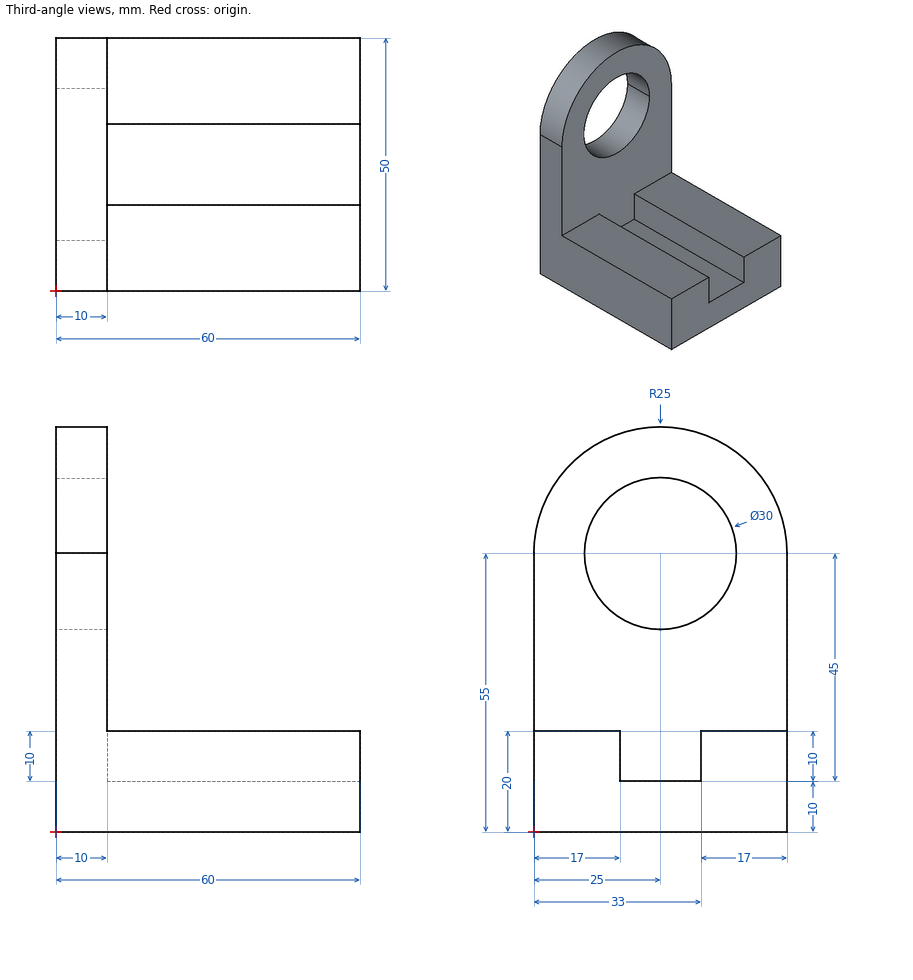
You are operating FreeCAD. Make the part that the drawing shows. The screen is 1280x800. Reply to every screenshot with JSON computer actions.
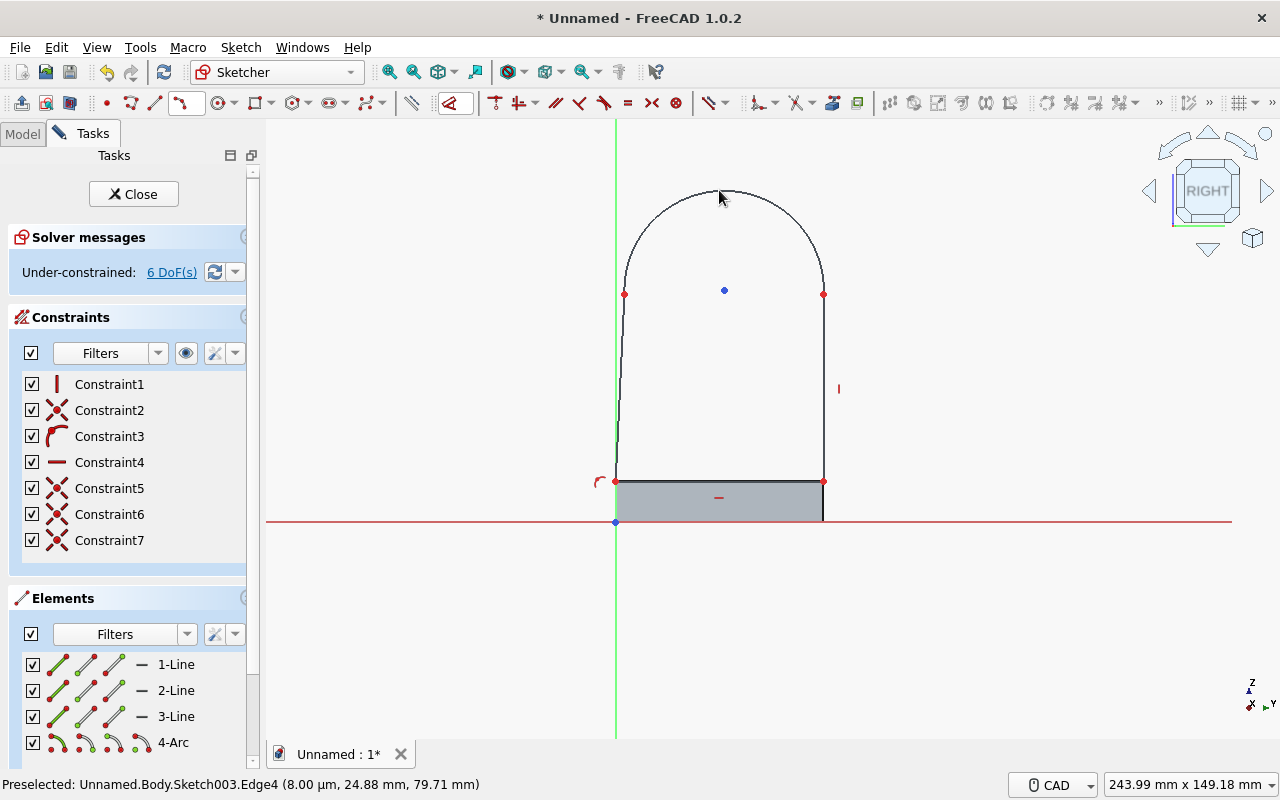
{"action": "left_click", "coordinate": [824, 351]}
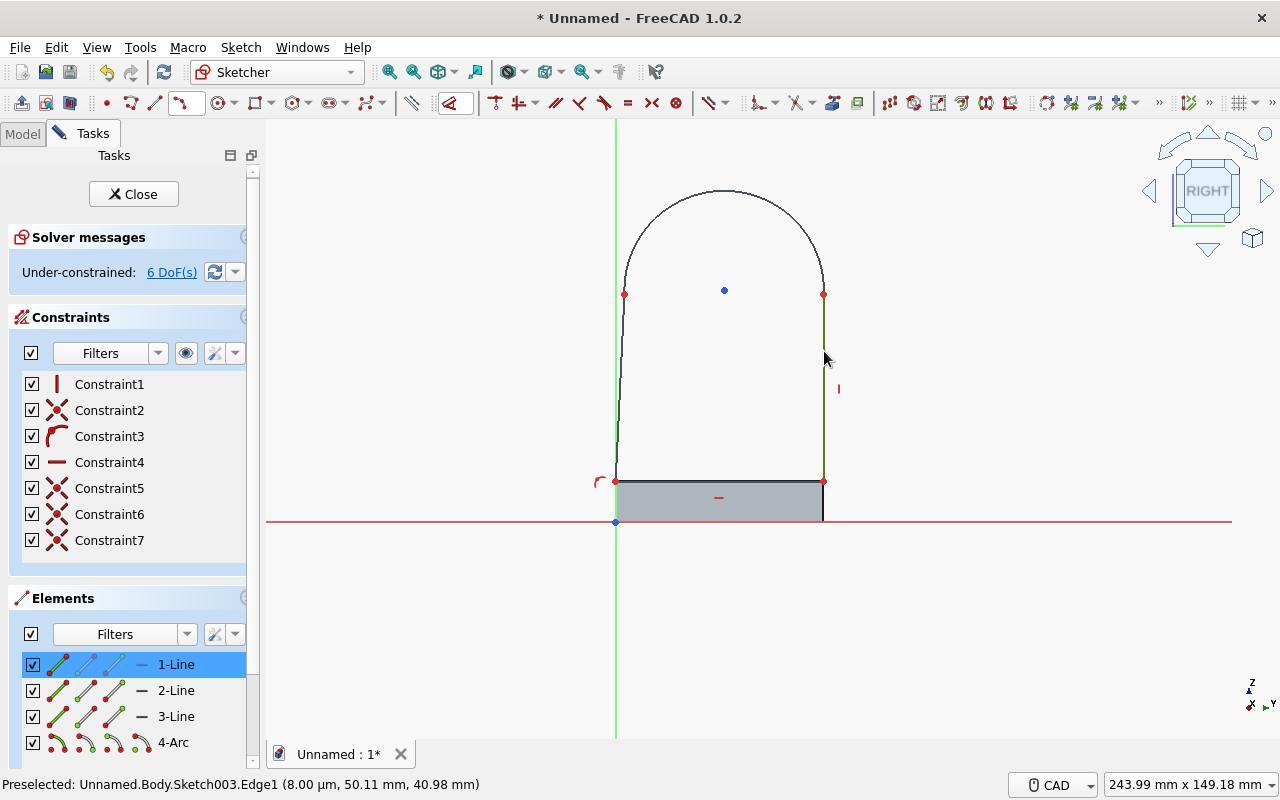
{"action": "left_click", "coordinate": [784, 211]}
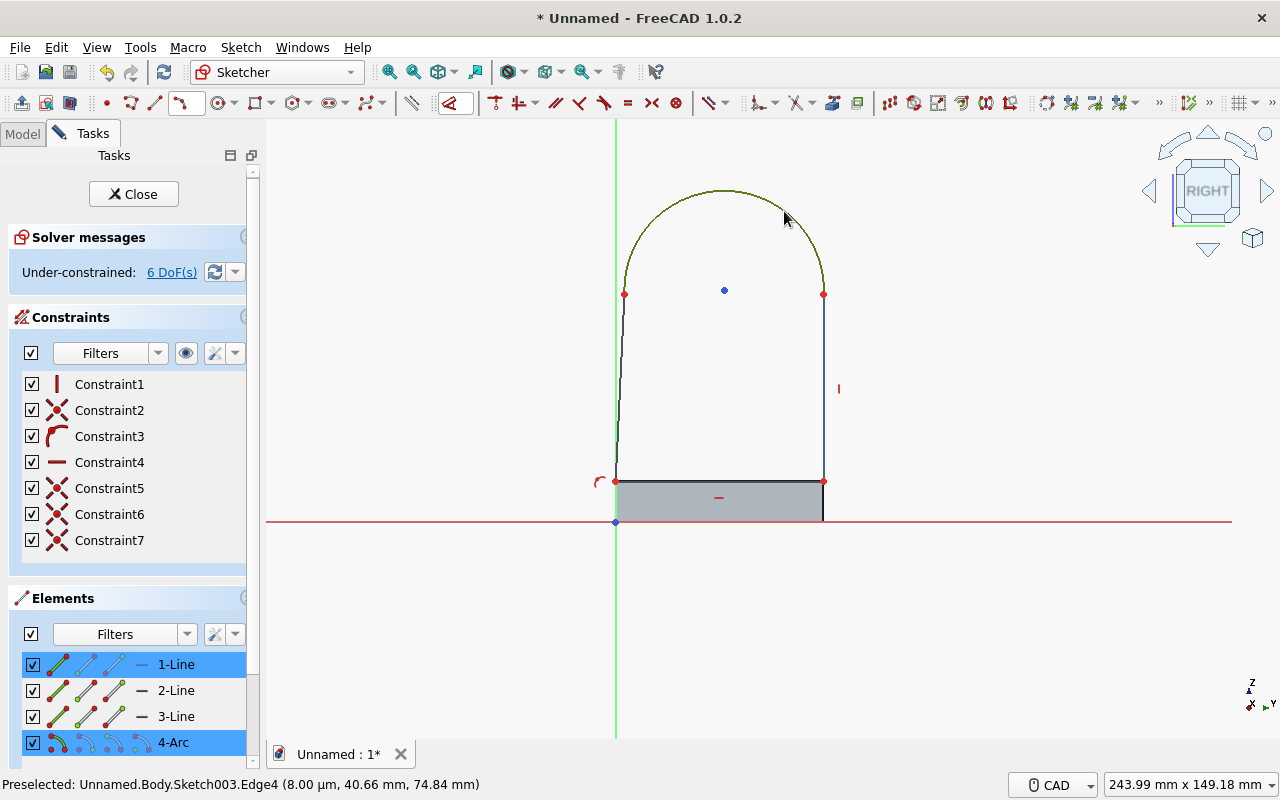
{"action": "left_click", "coordinate": [604, 104]}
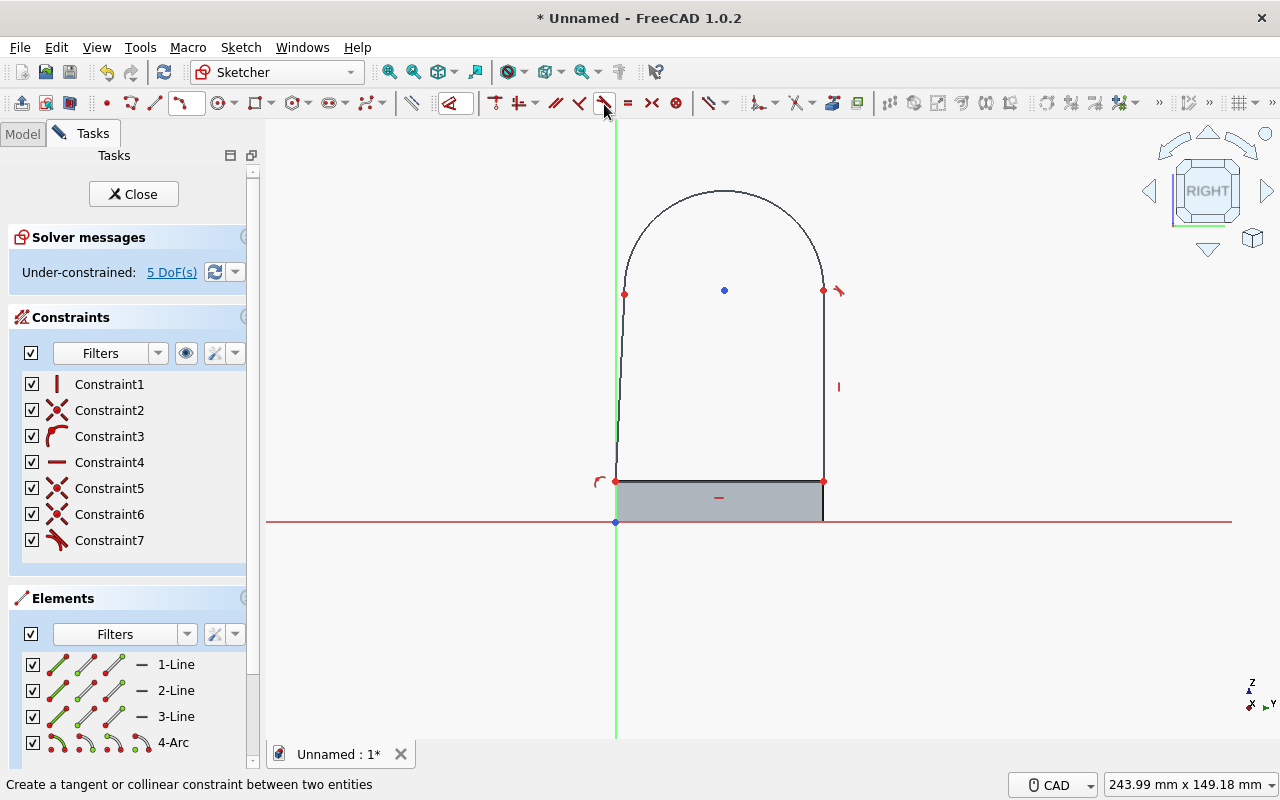
{"action": "left_click", "coordinate": [618, 426]}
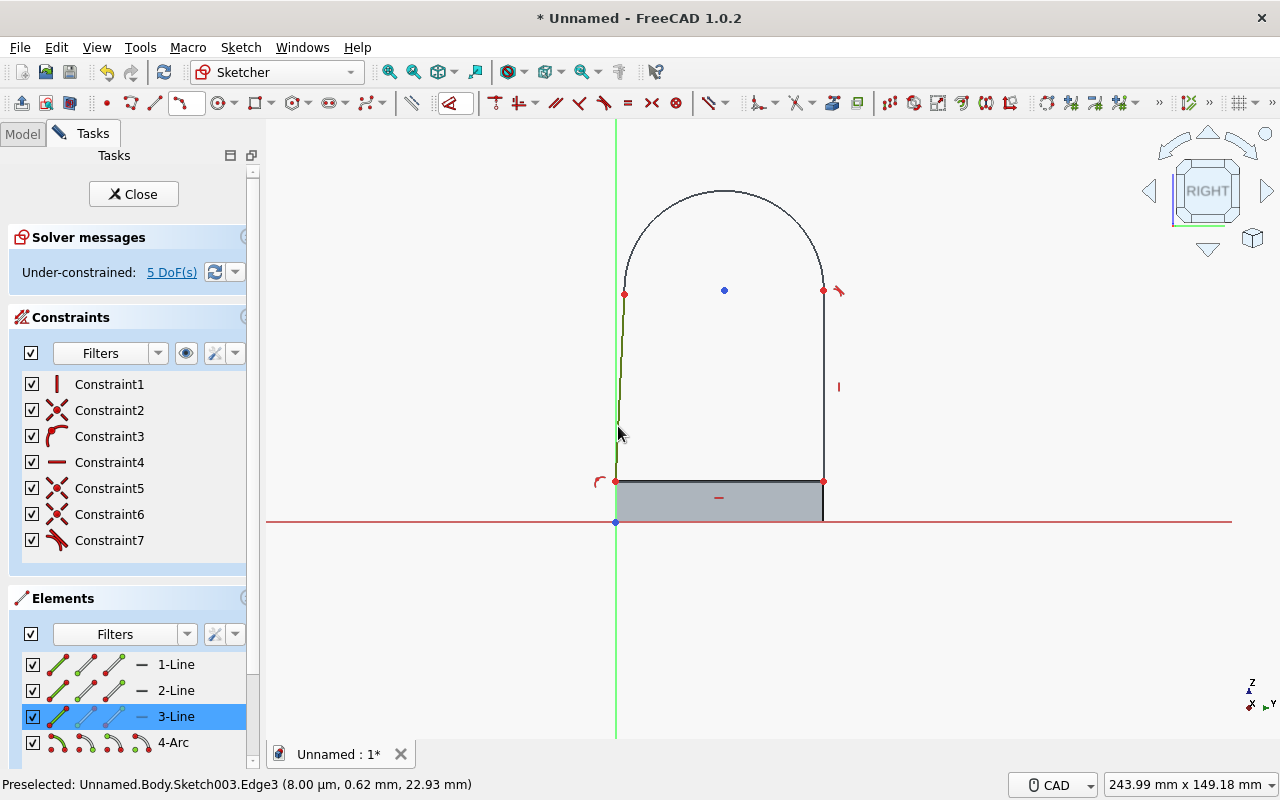
{"action": "left_click", "coordinate": [782, 209]}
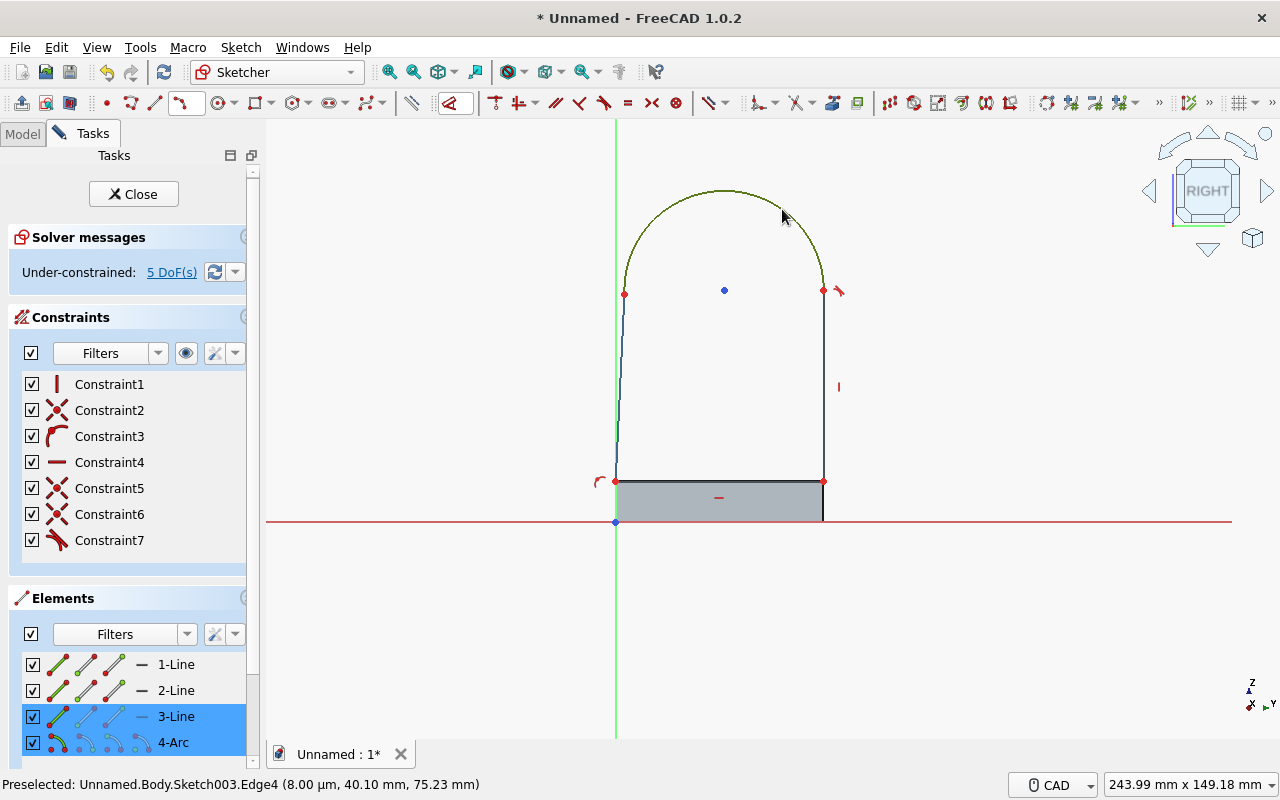
{"action": "left_click", "coordinate": [604, 104]}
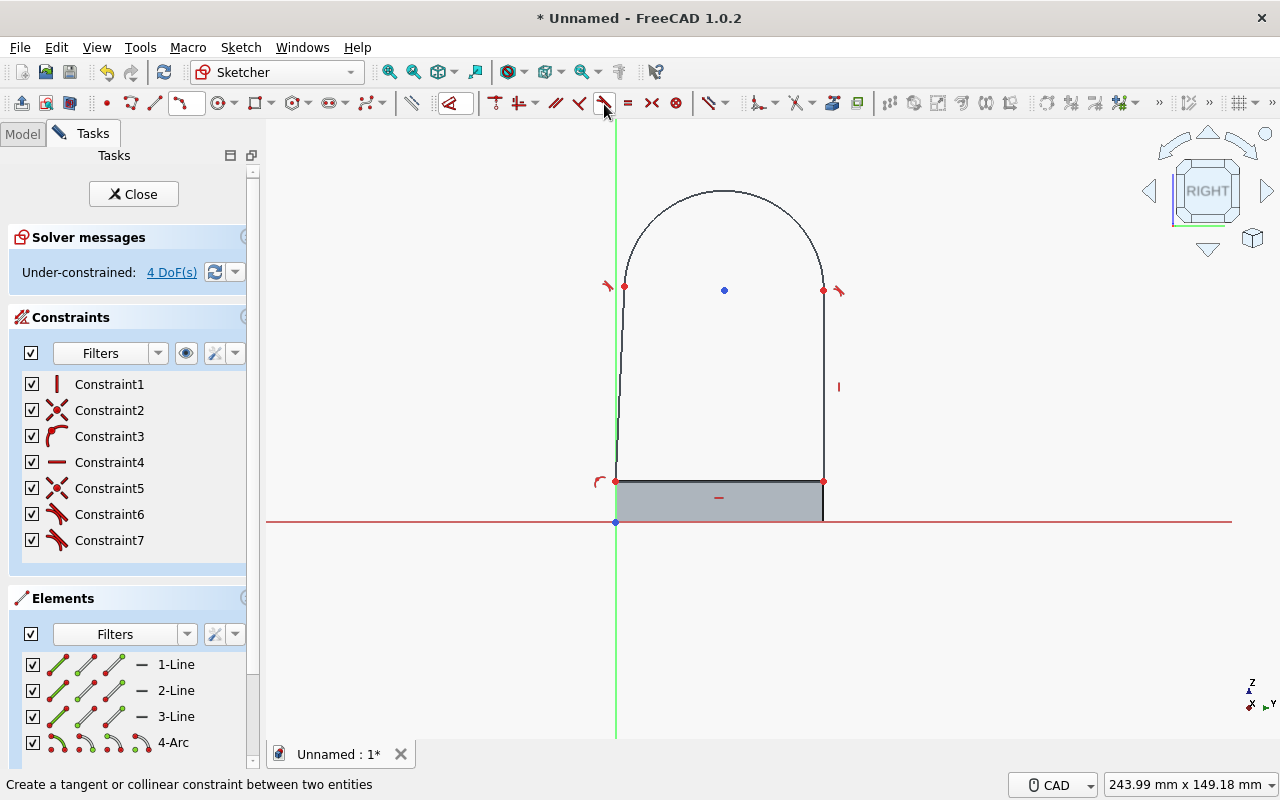
{"action": "left_click", "coordinate": [618, 423]}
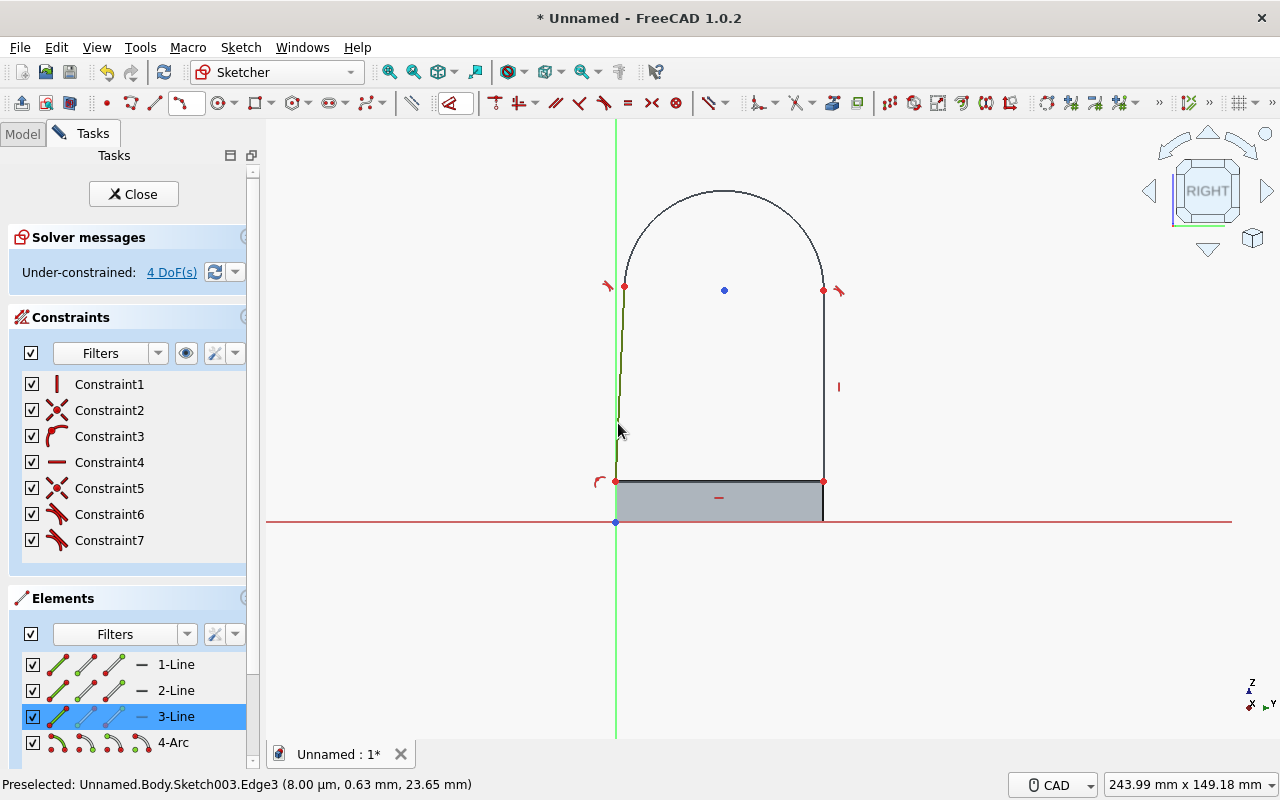
{"action": "key", "text": "v"}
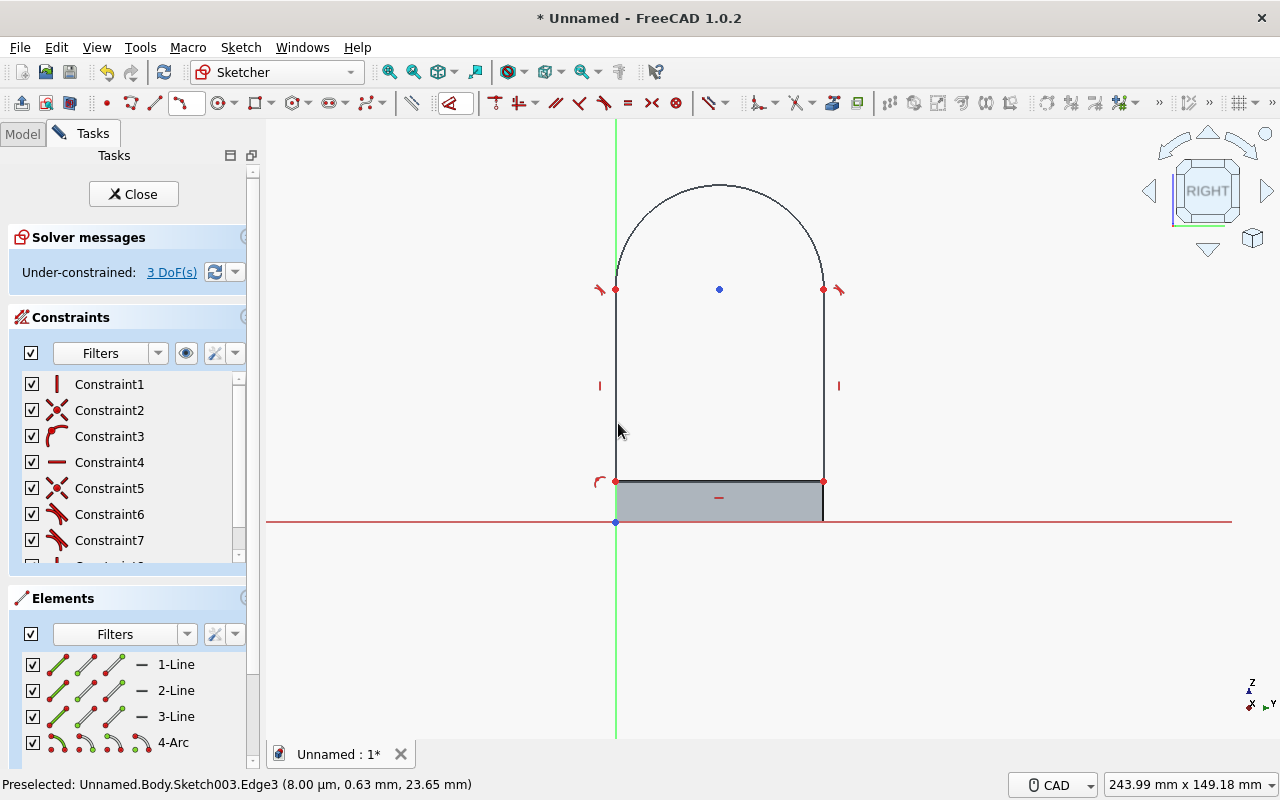
{"action": "left_click", "coordinate": [781, 205]}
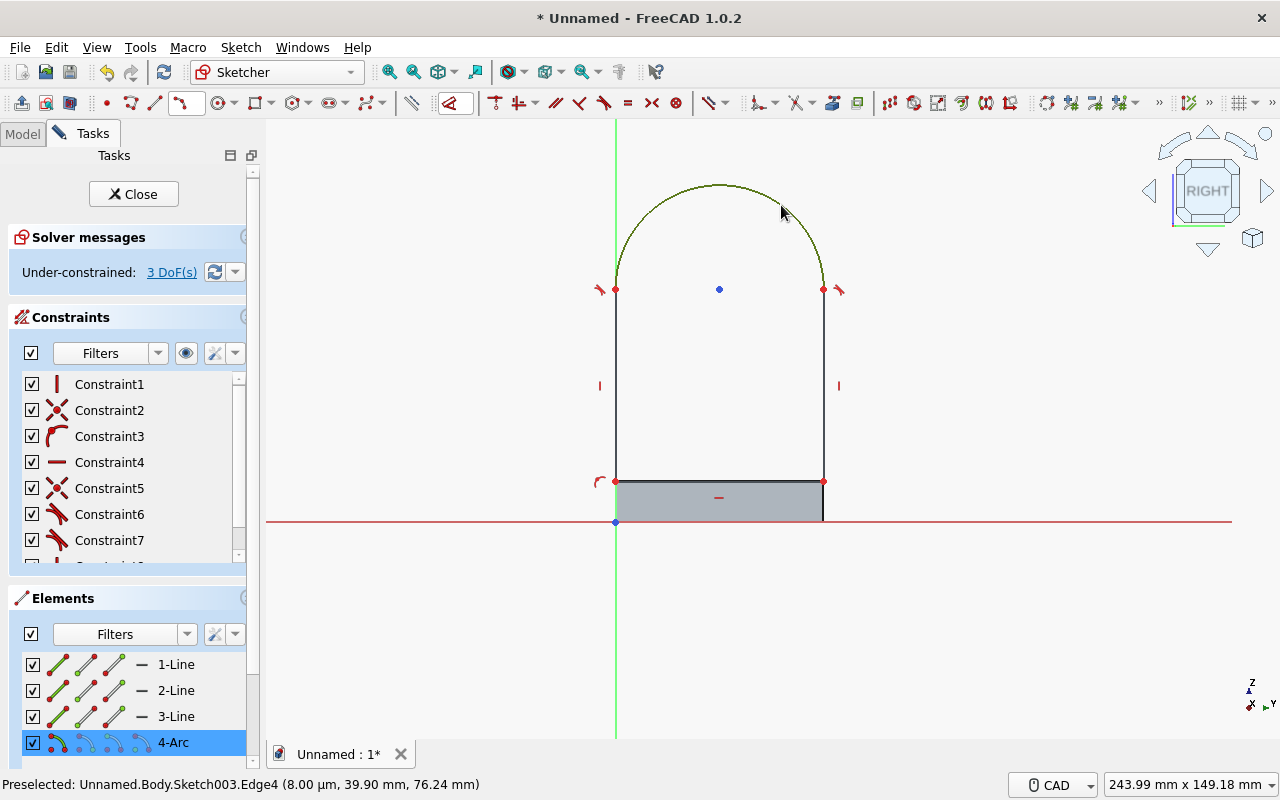
{"action": "left_click", "coordinate": [468, 104]}